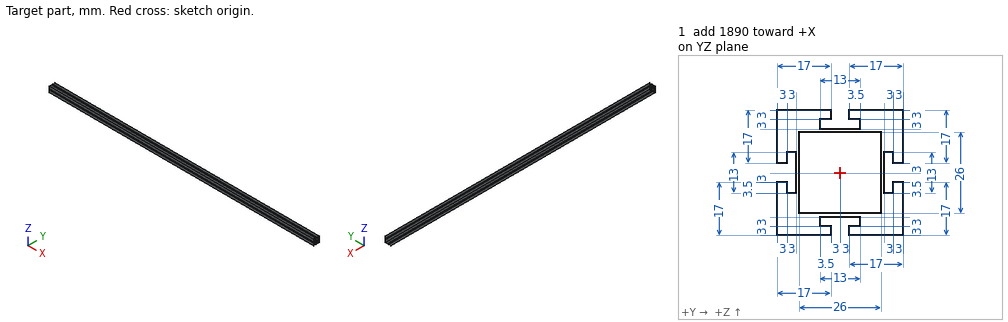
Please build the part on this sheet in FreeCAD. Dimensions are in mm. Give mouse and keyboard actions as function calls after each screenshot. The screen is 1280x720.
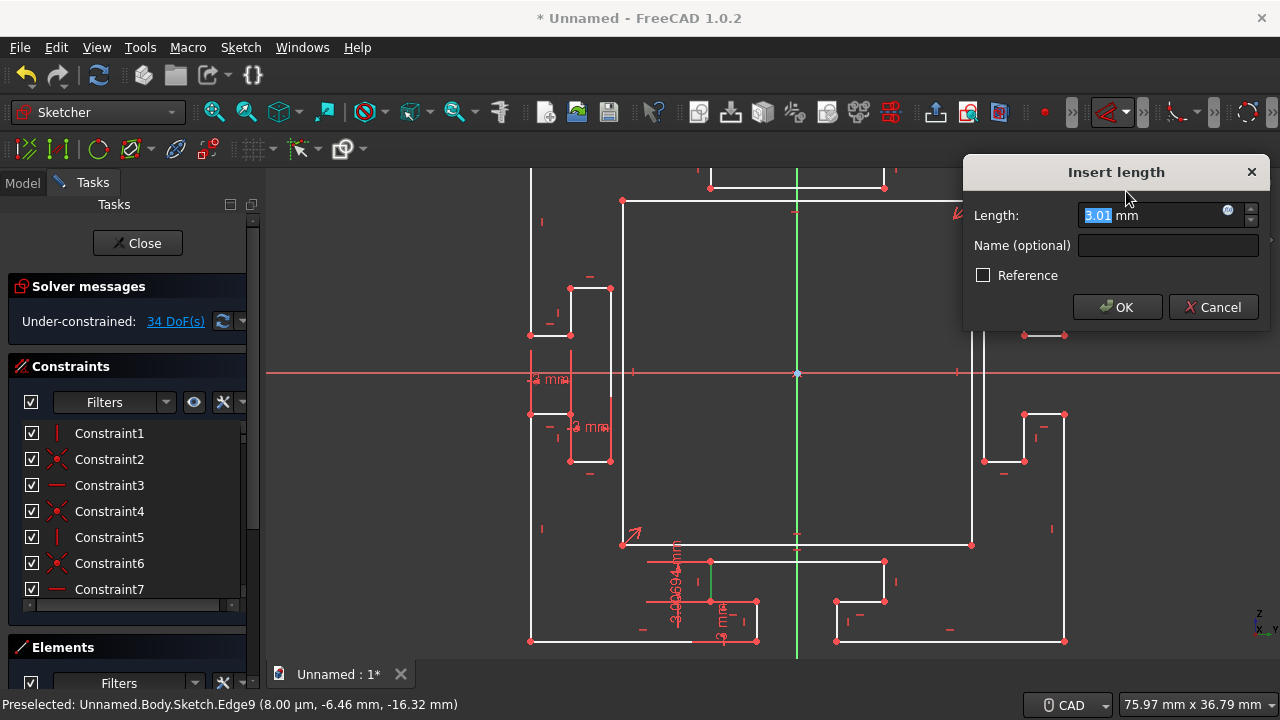
text(3)
key(Return)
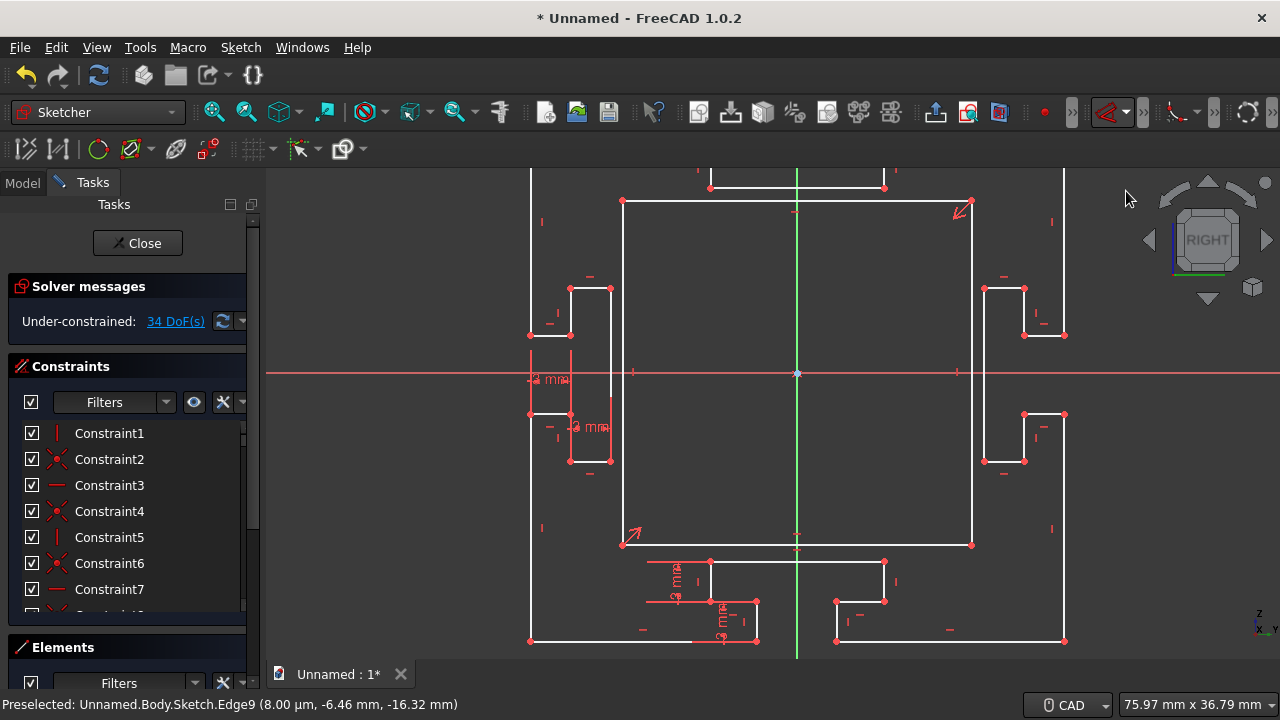
click(884, 574)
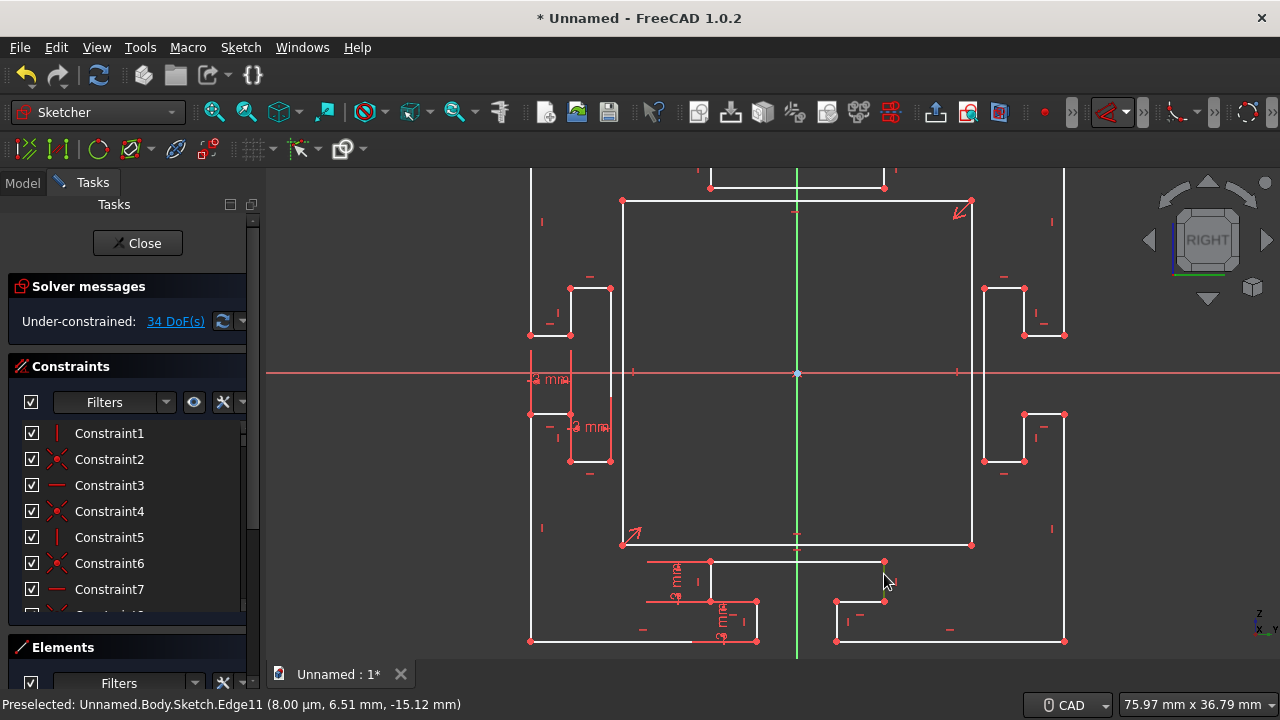
key(i)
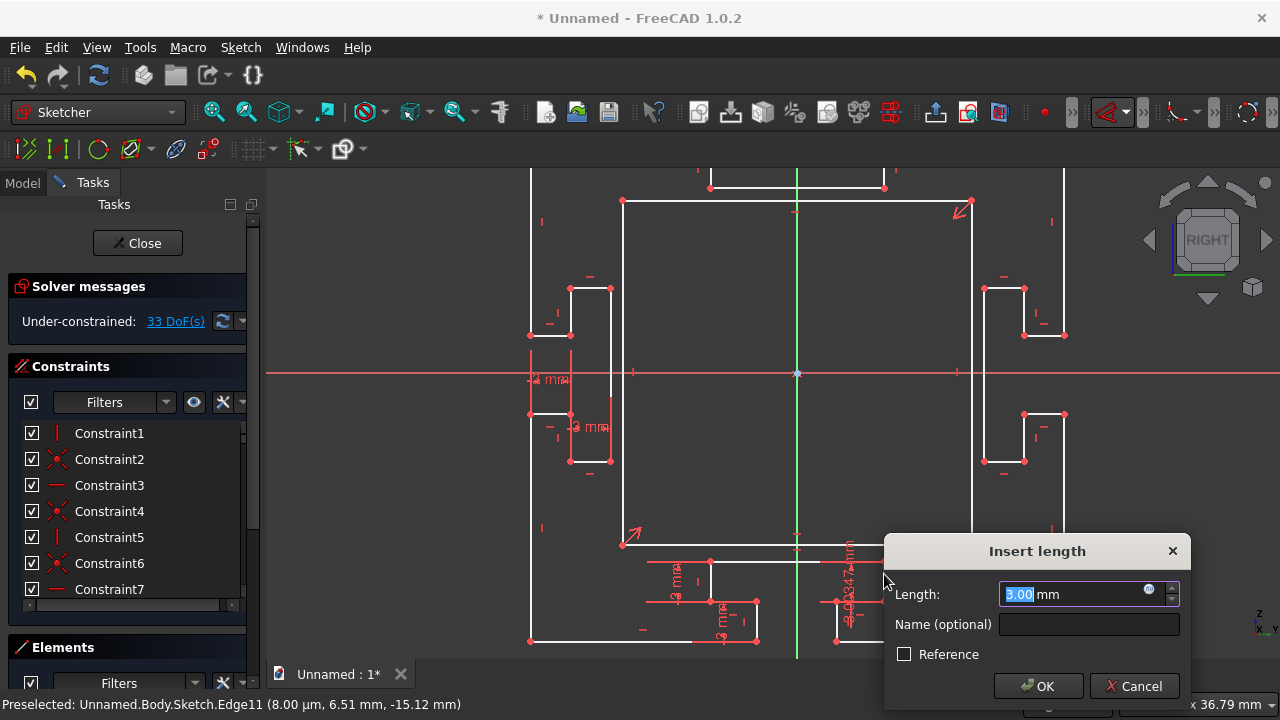
text(3)
key(Return)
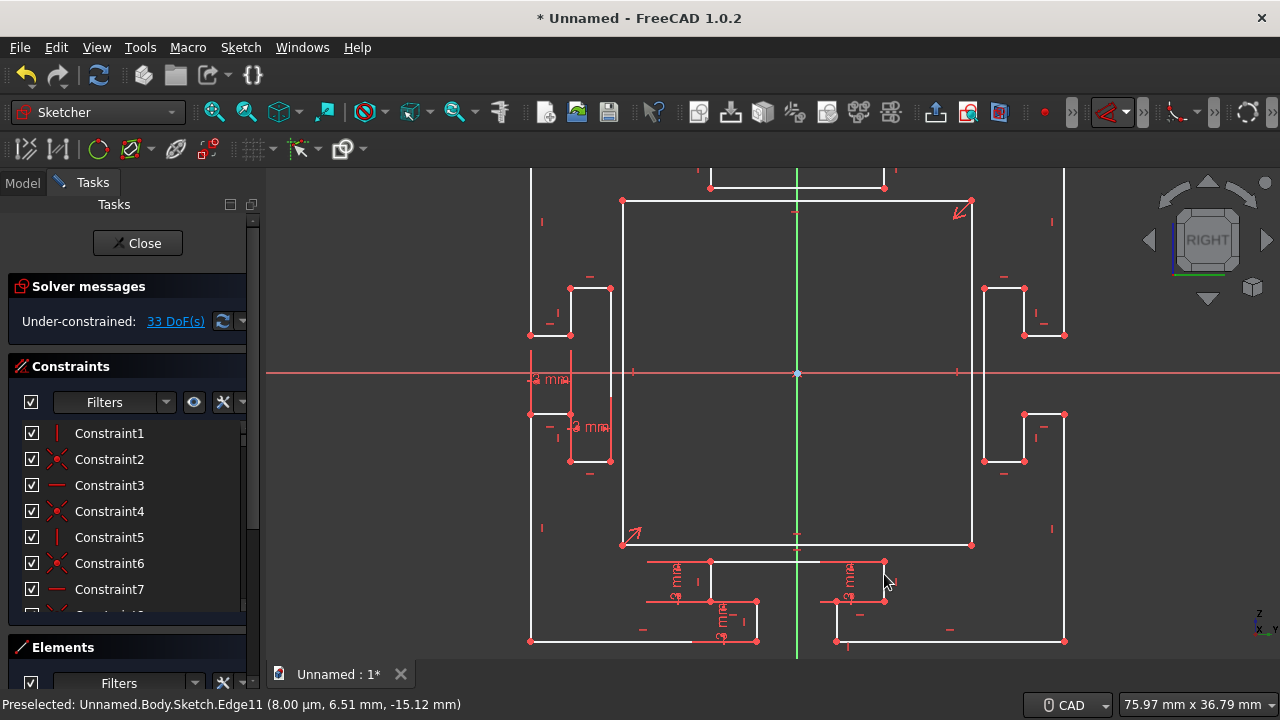
click(837, 614)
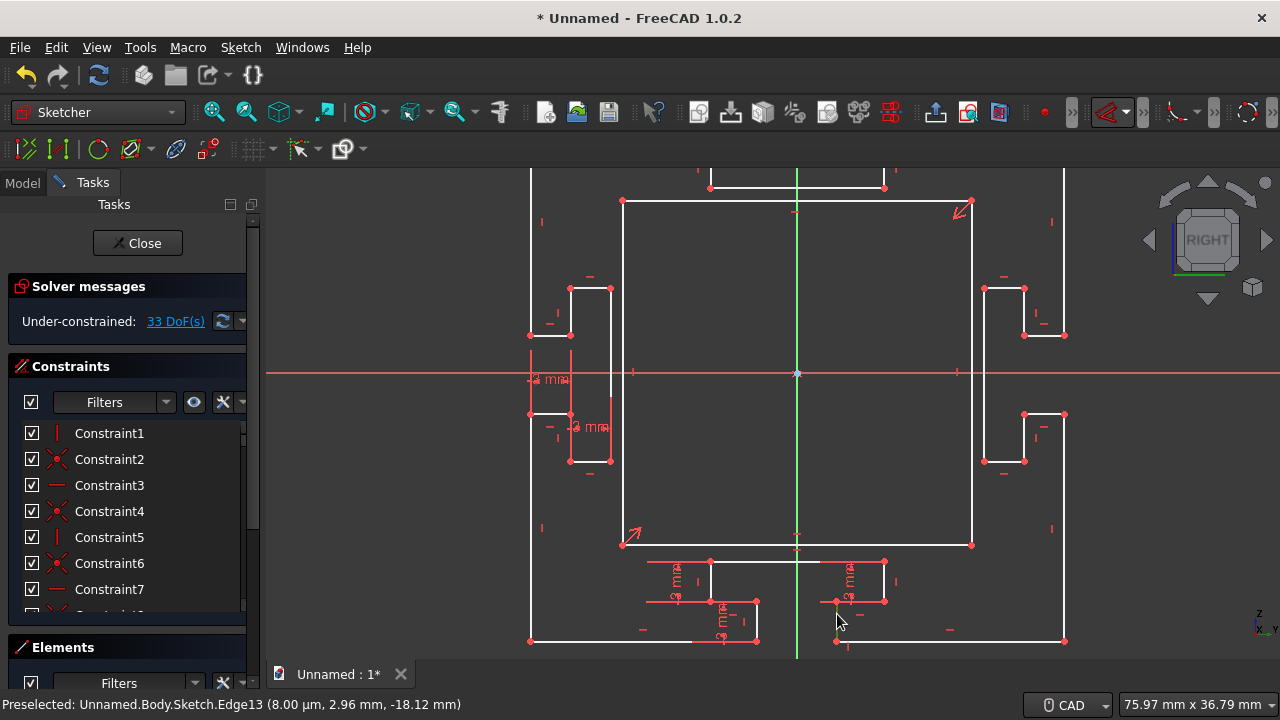
key(i)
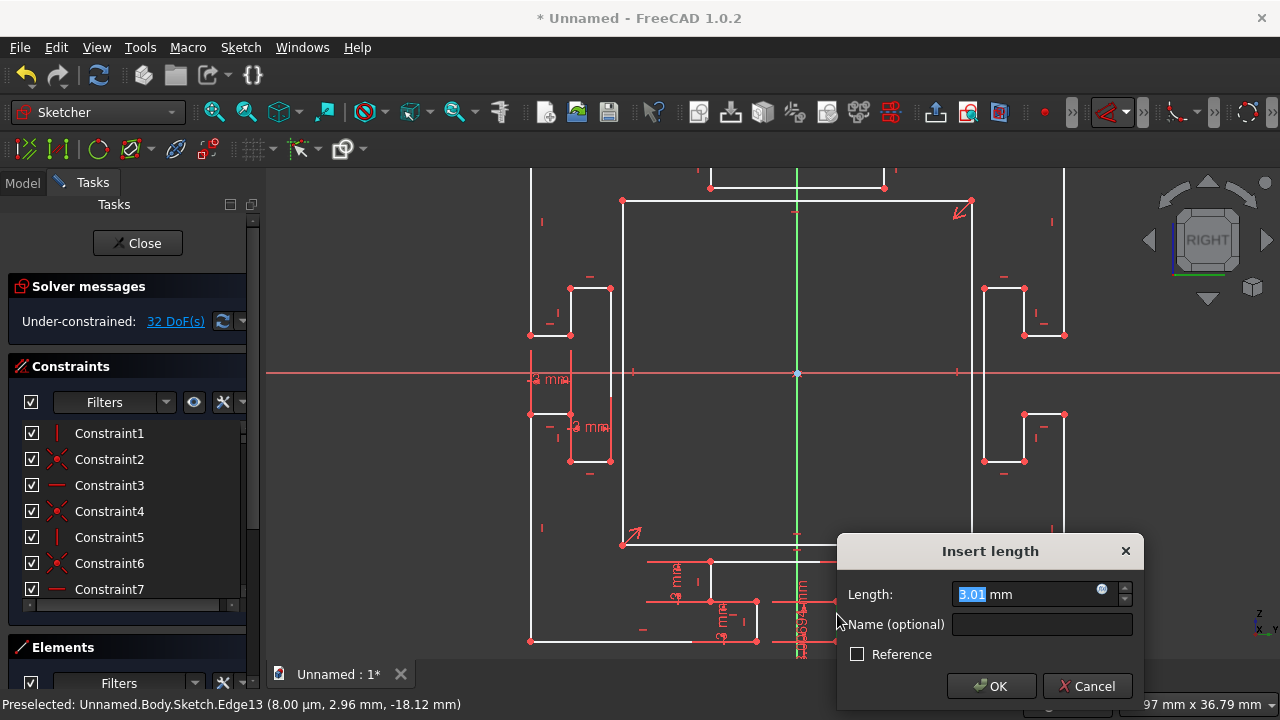
text(3)
key(Return)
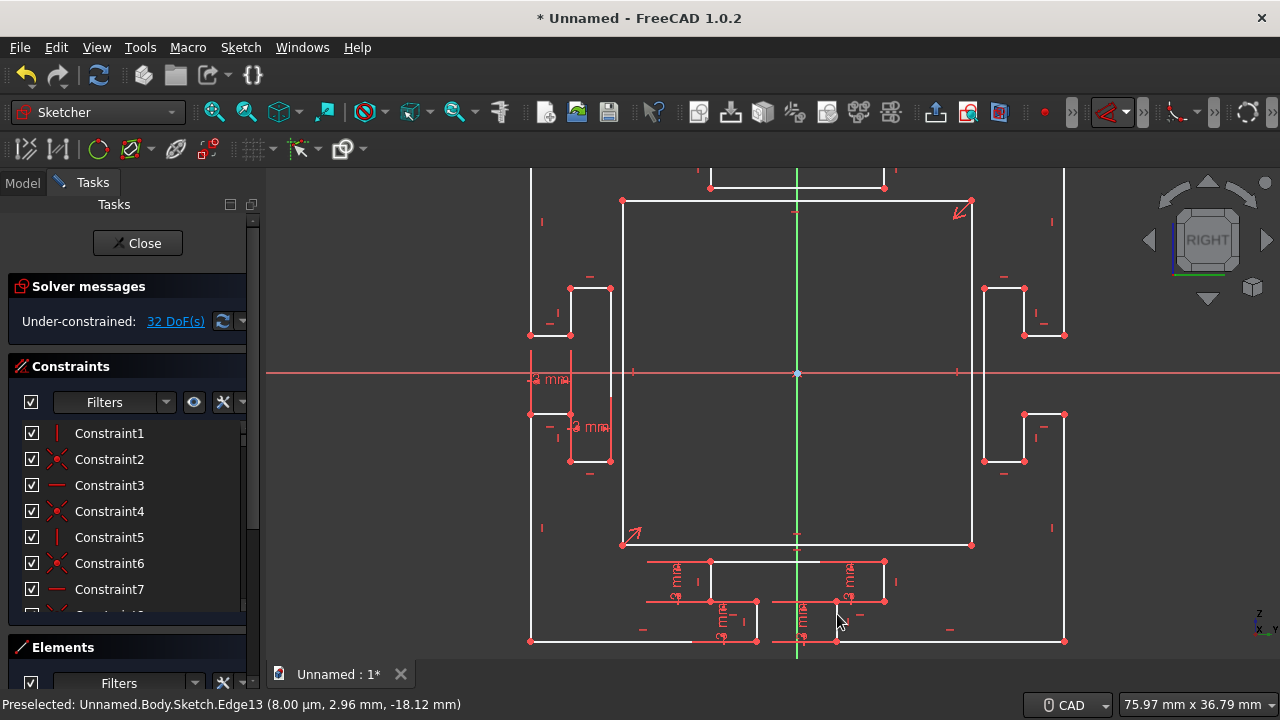
click(1052, 414)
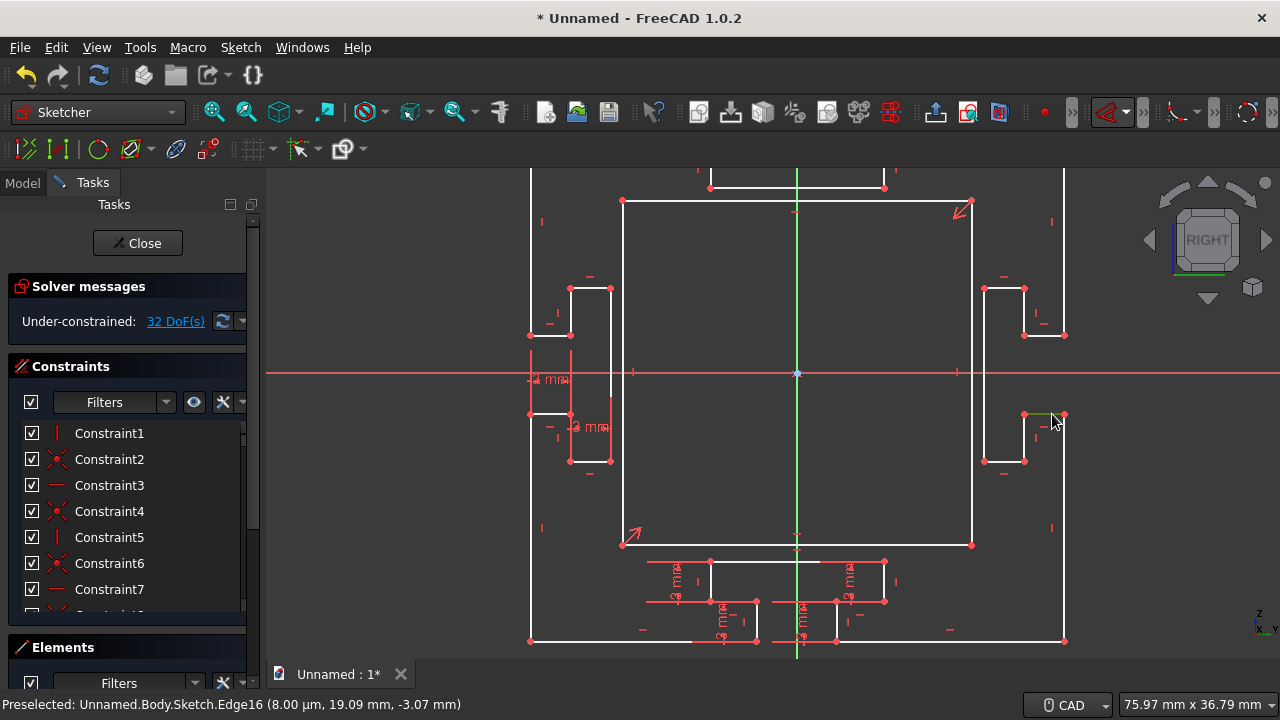
key(l)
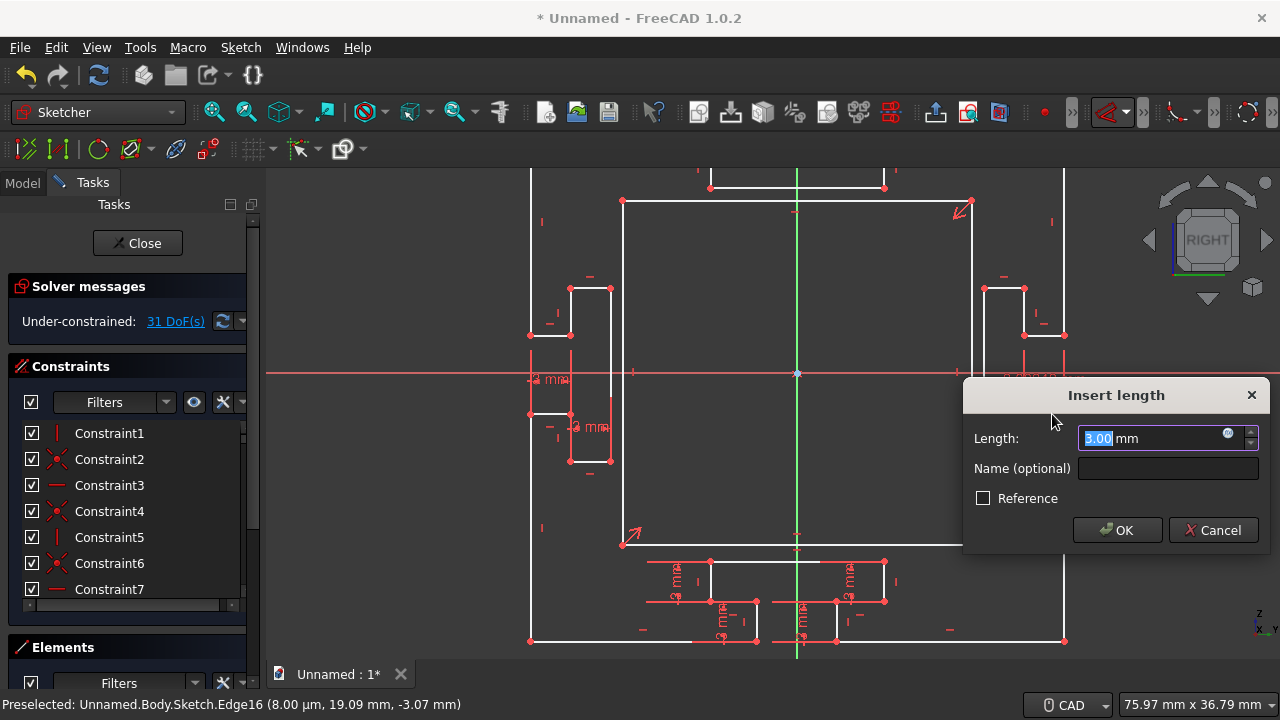
text(3)
key(Return)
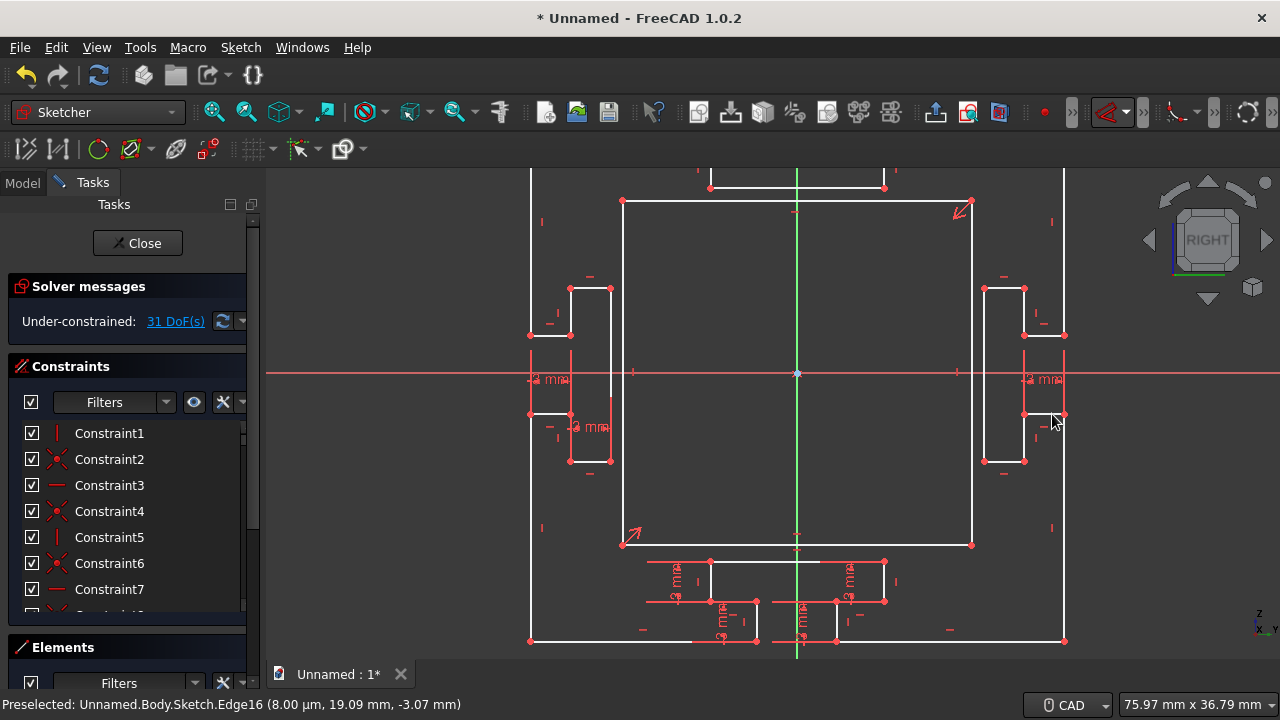
click(1012, 462)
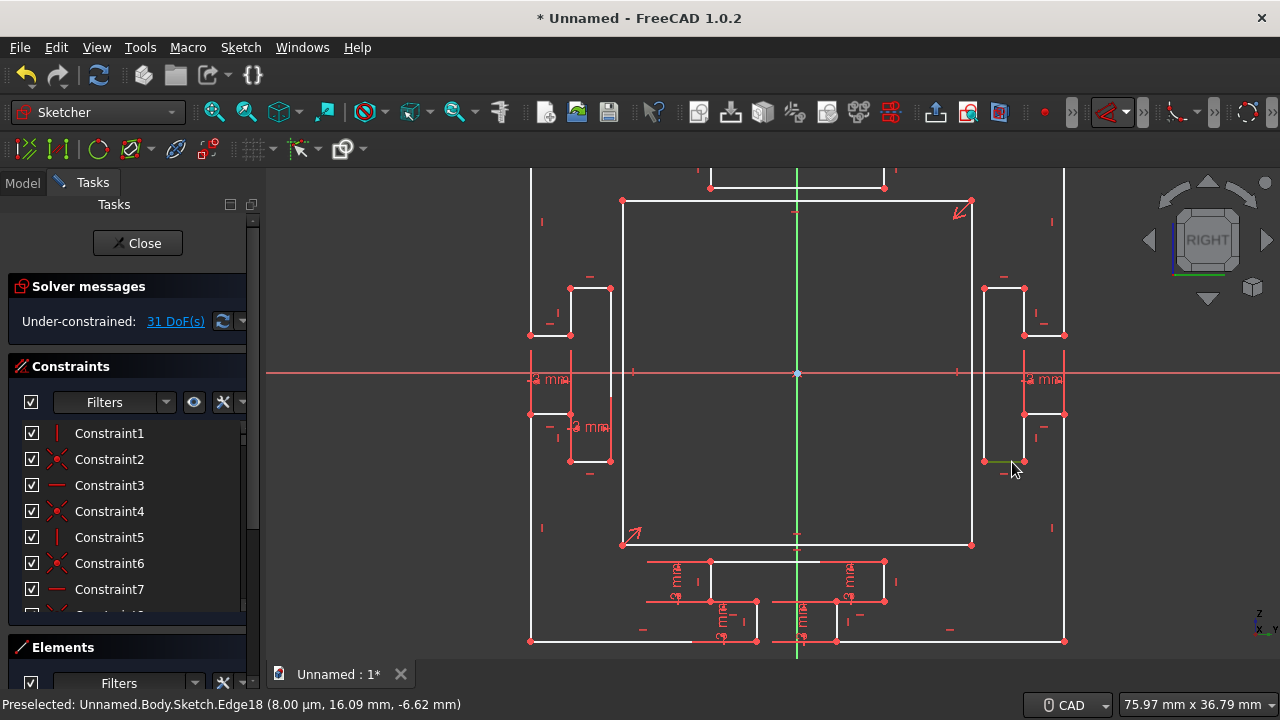
key(l)